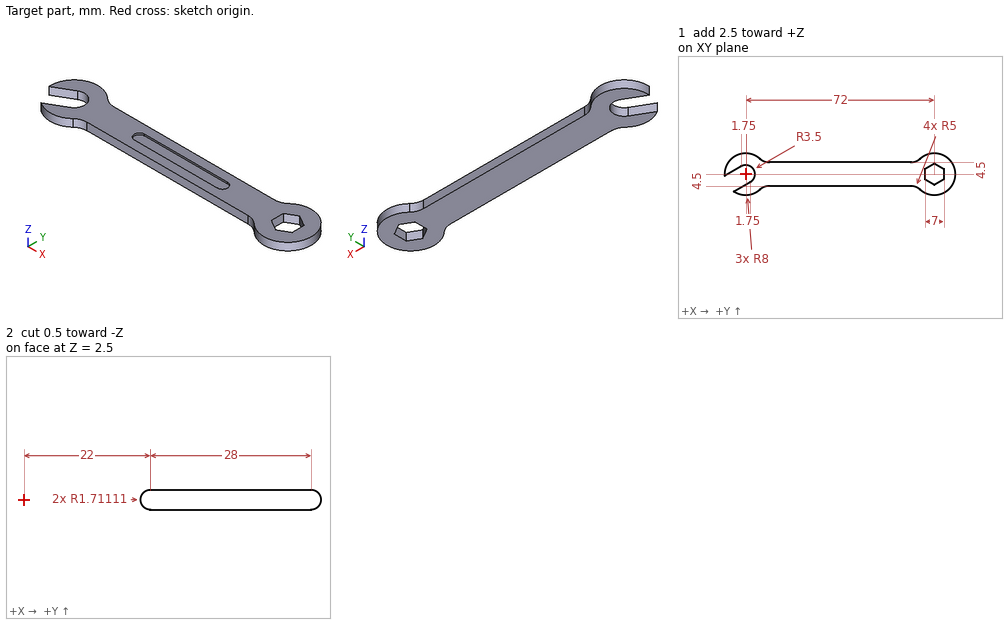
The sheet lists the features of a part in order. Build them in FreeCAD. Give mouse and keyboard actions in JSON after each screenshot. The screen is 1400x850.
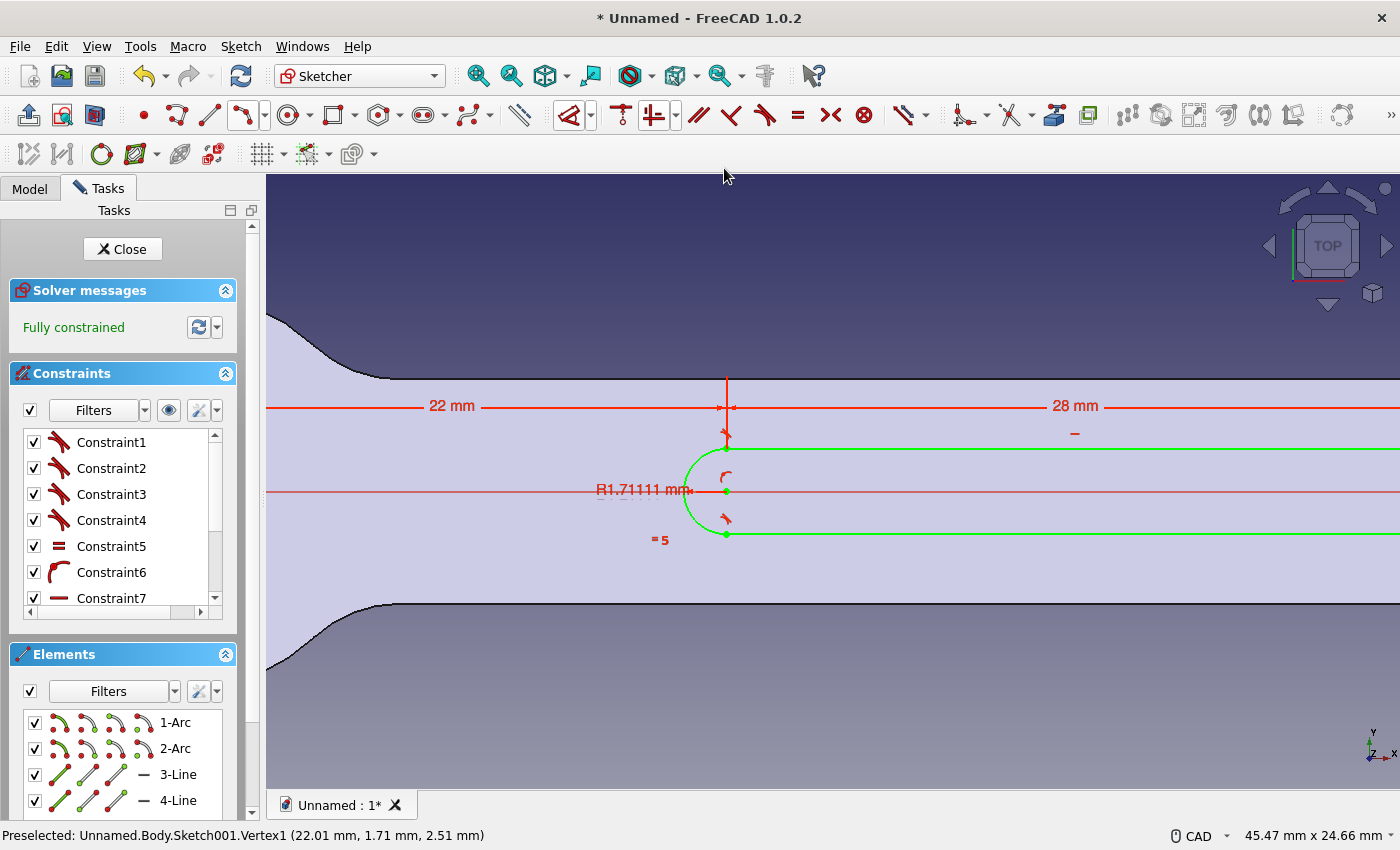
{"action": "left_click", "coordinate": [123, 249]}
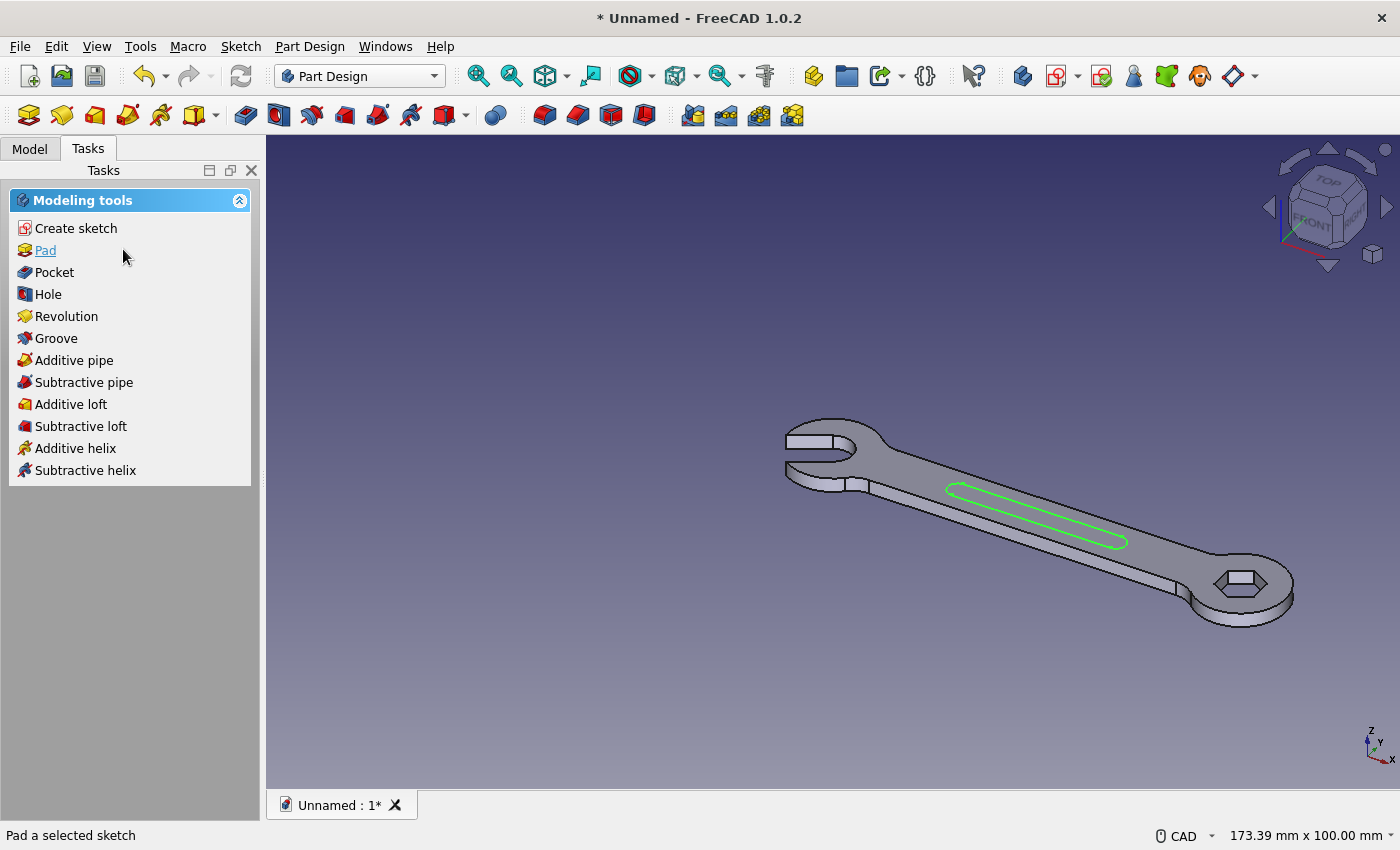
{"action": "left_click", "coordinate": [246, 116]}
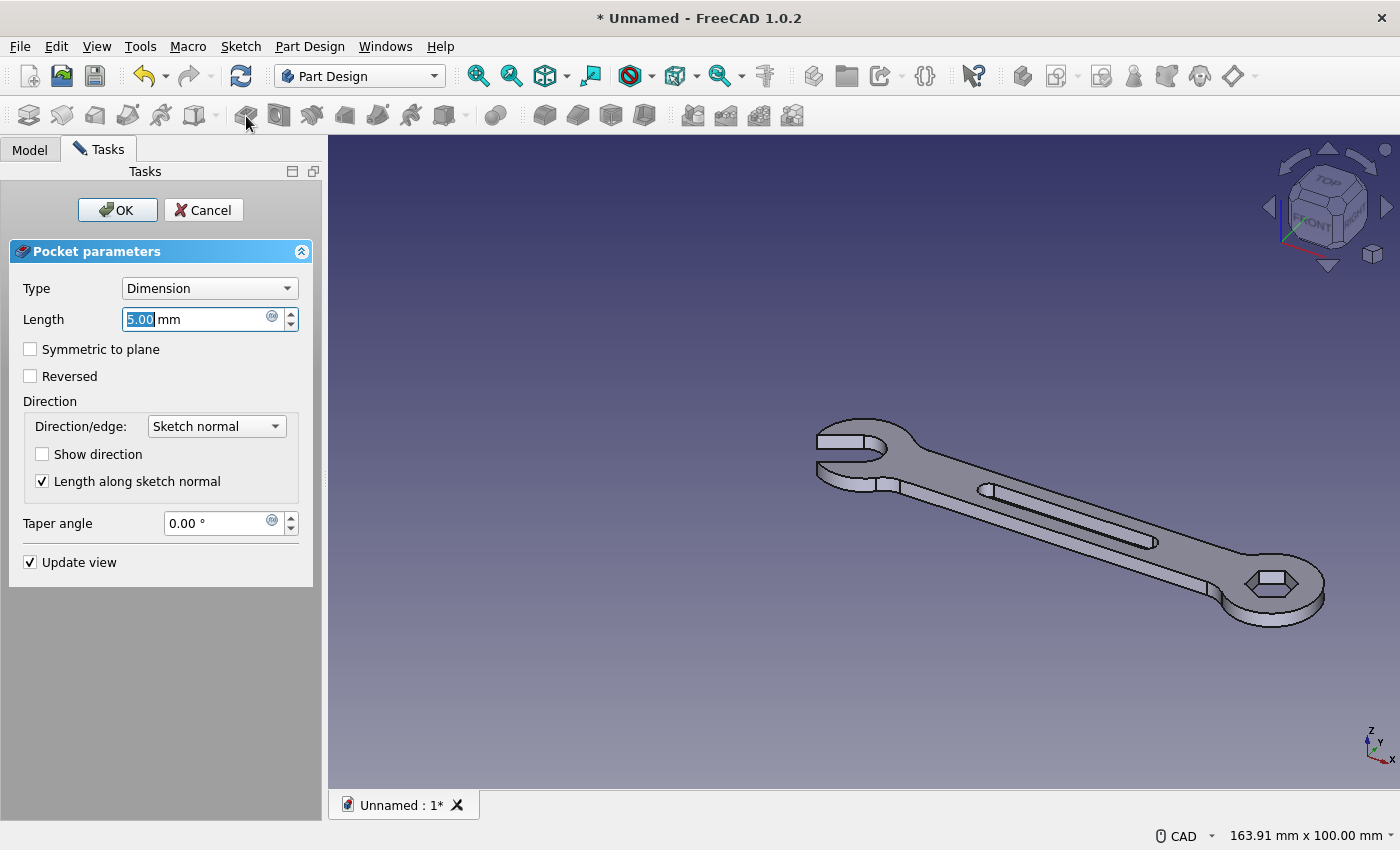
{"action": "type", "text": "0.5"}
{"action": "key", "text": "Tab"}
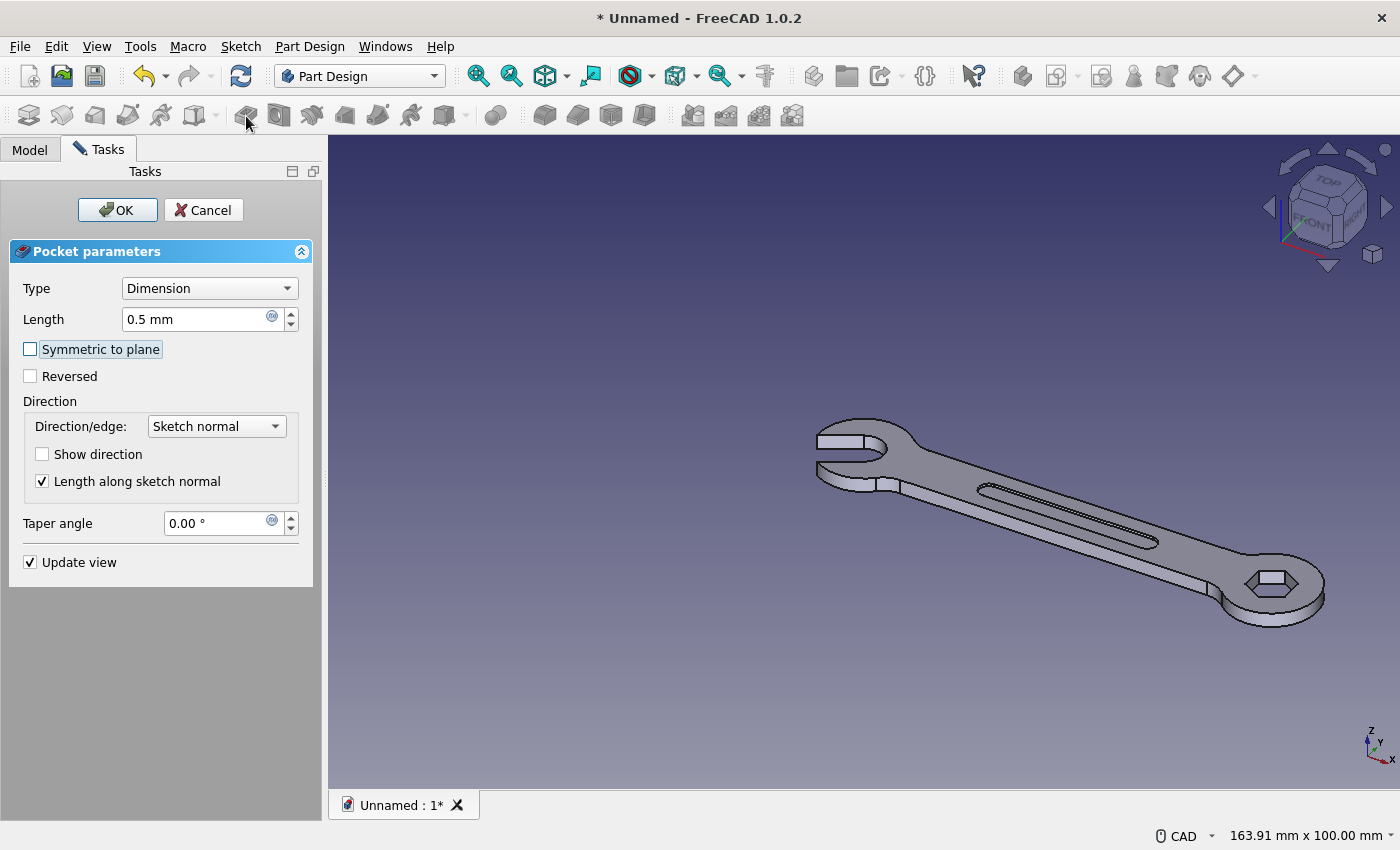
{"action": "left_click", "coordinate": [118, 210]}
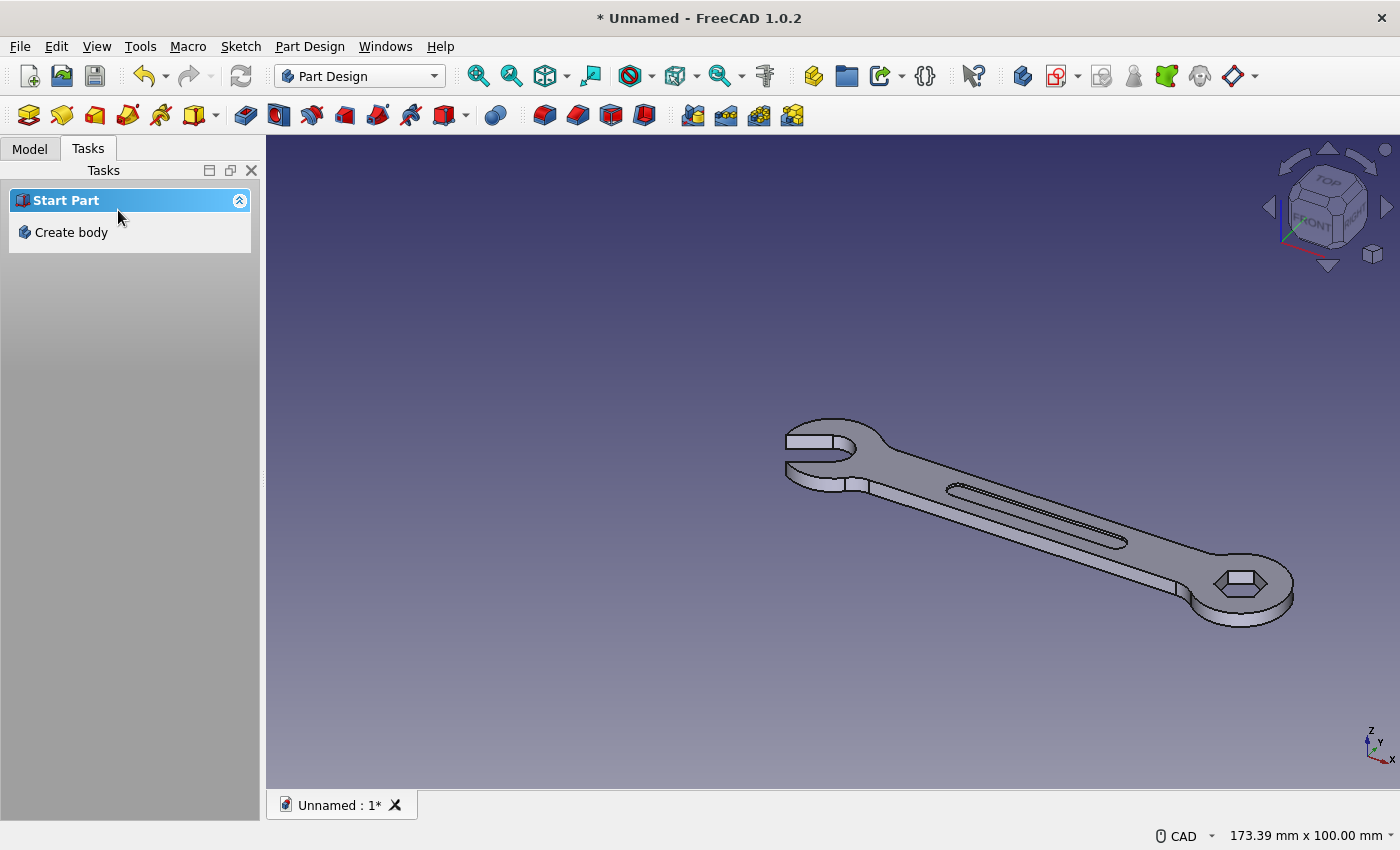
{"action": "key", "text": "0"}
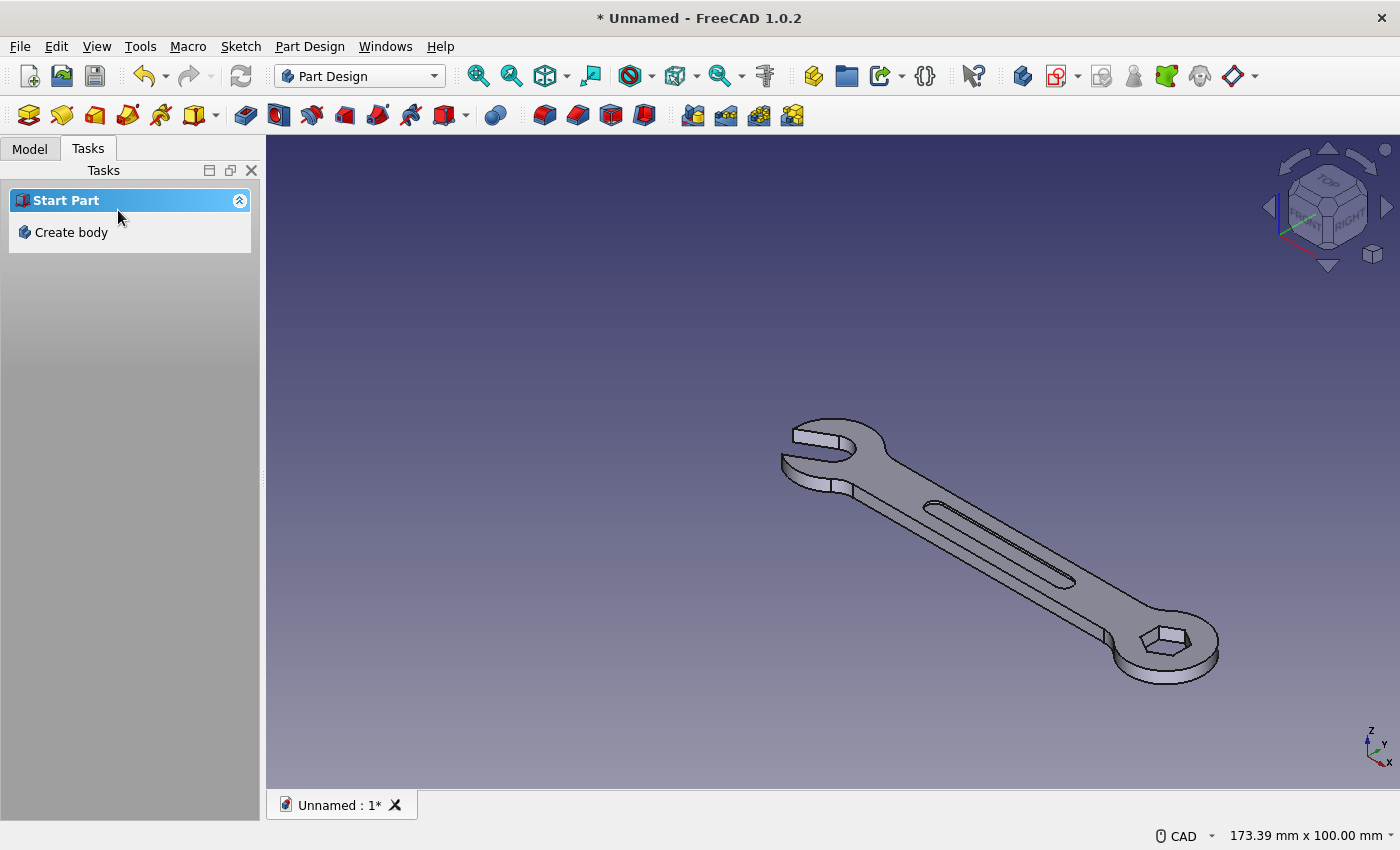
{"action": "left_click", "coordinate": [479, 76]}